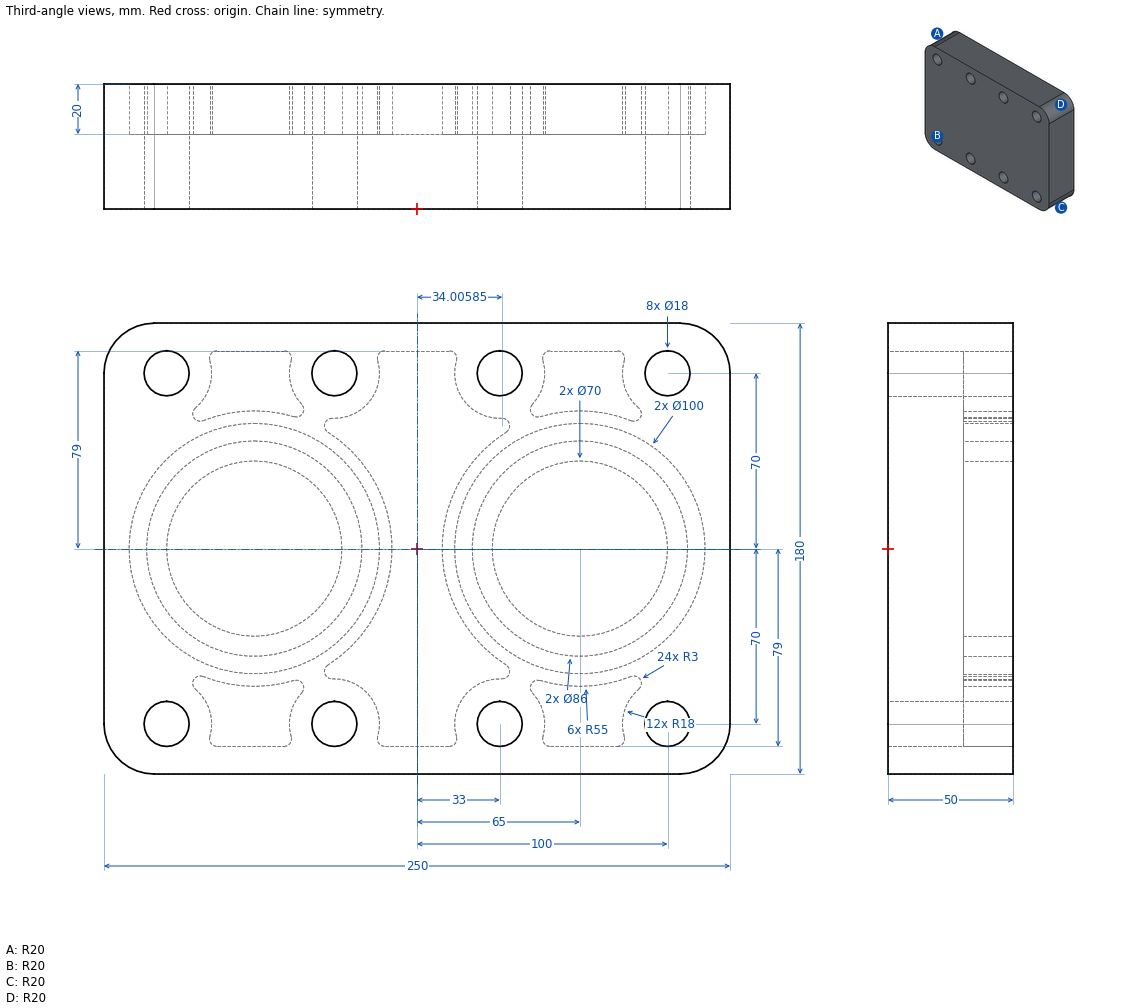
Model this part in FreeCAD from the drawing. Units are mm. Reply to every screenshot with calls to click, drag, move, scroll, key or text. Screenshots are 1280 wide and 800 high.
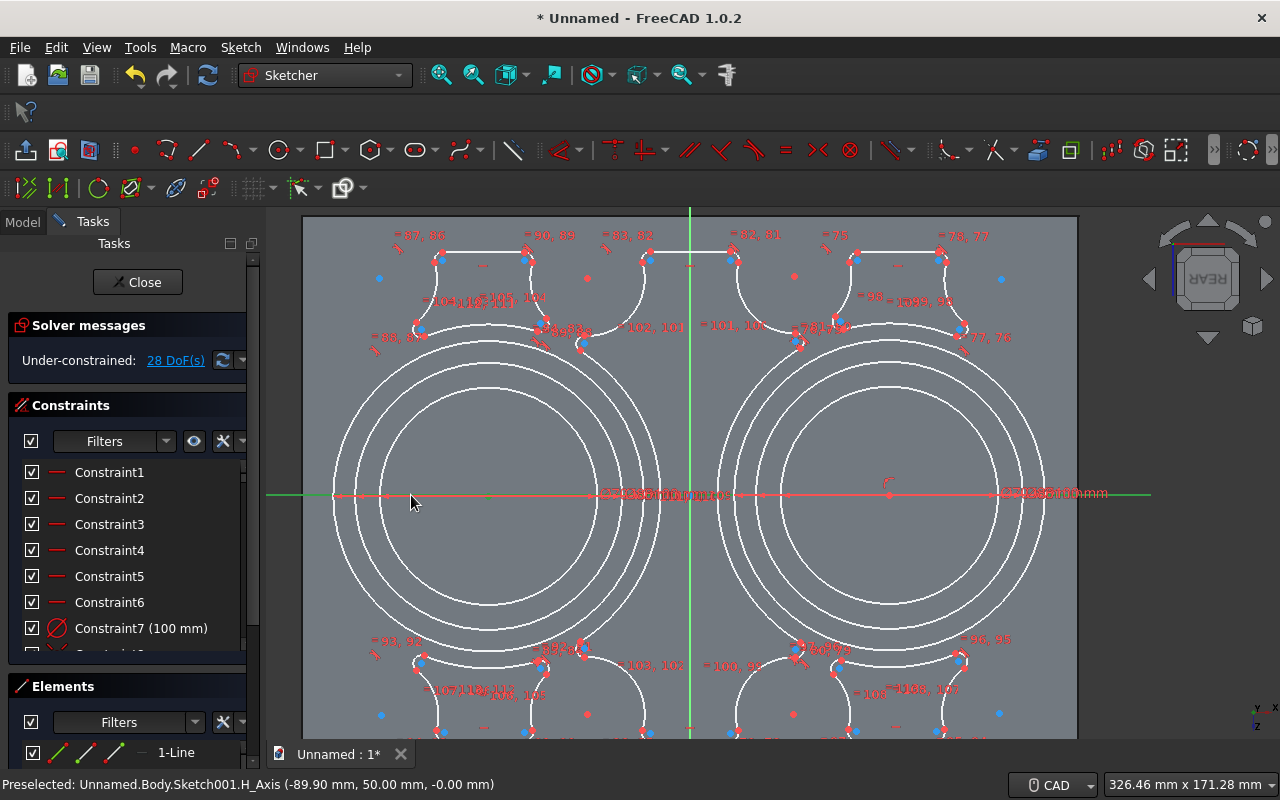
click(614, 150)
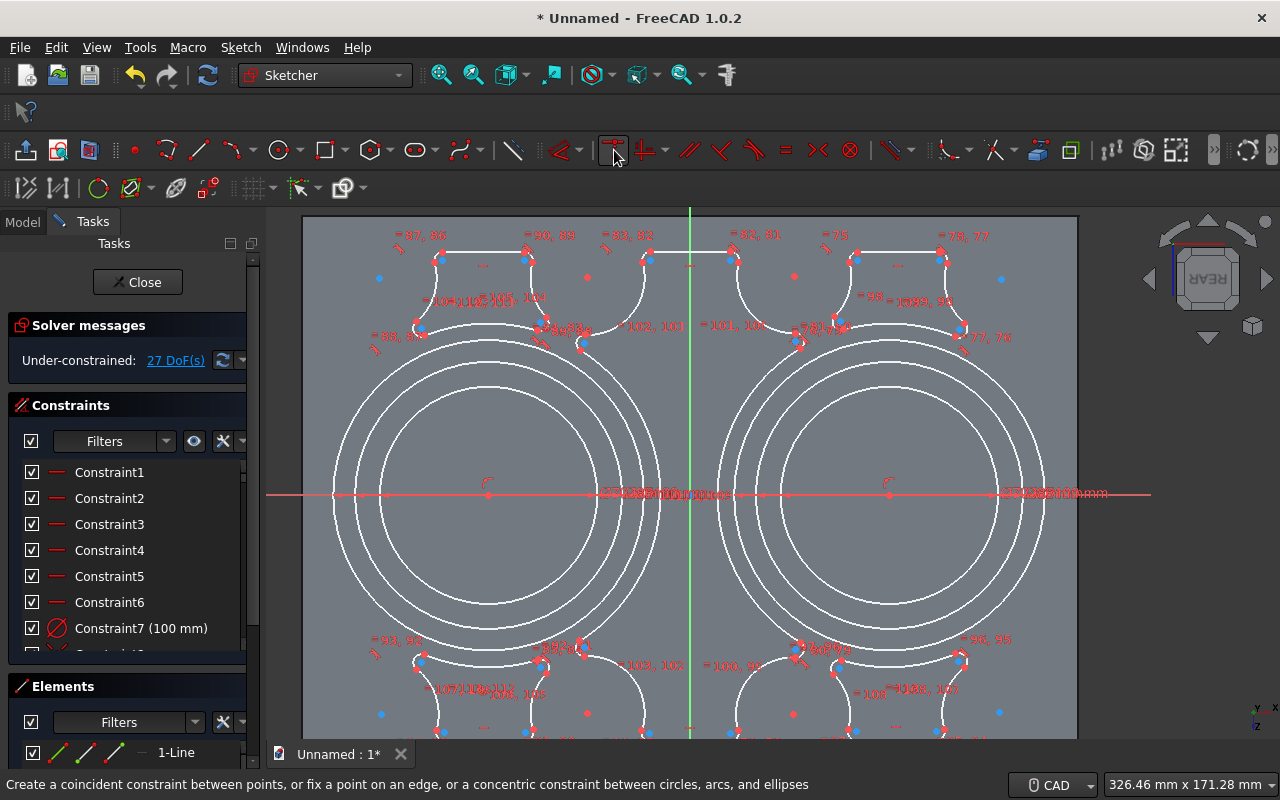
click(794, 276)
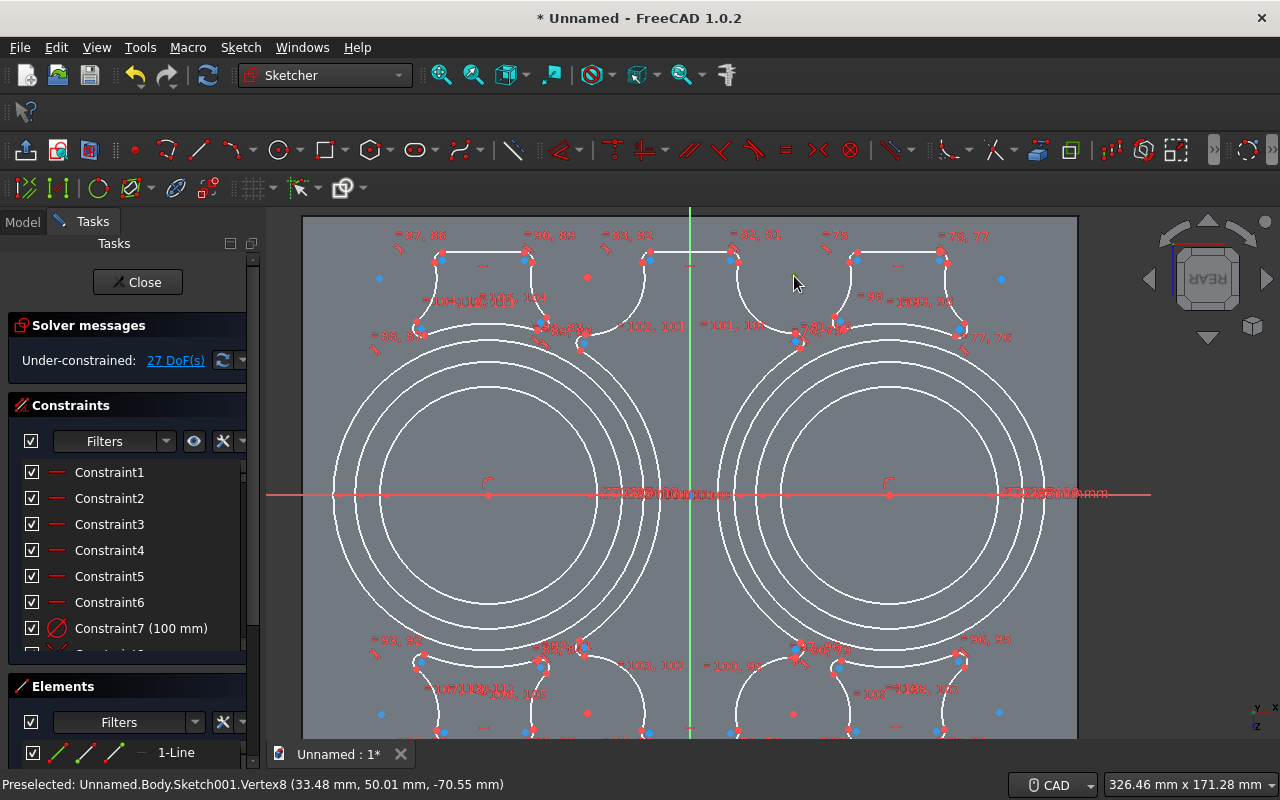
scroll(733, 427, down, 2)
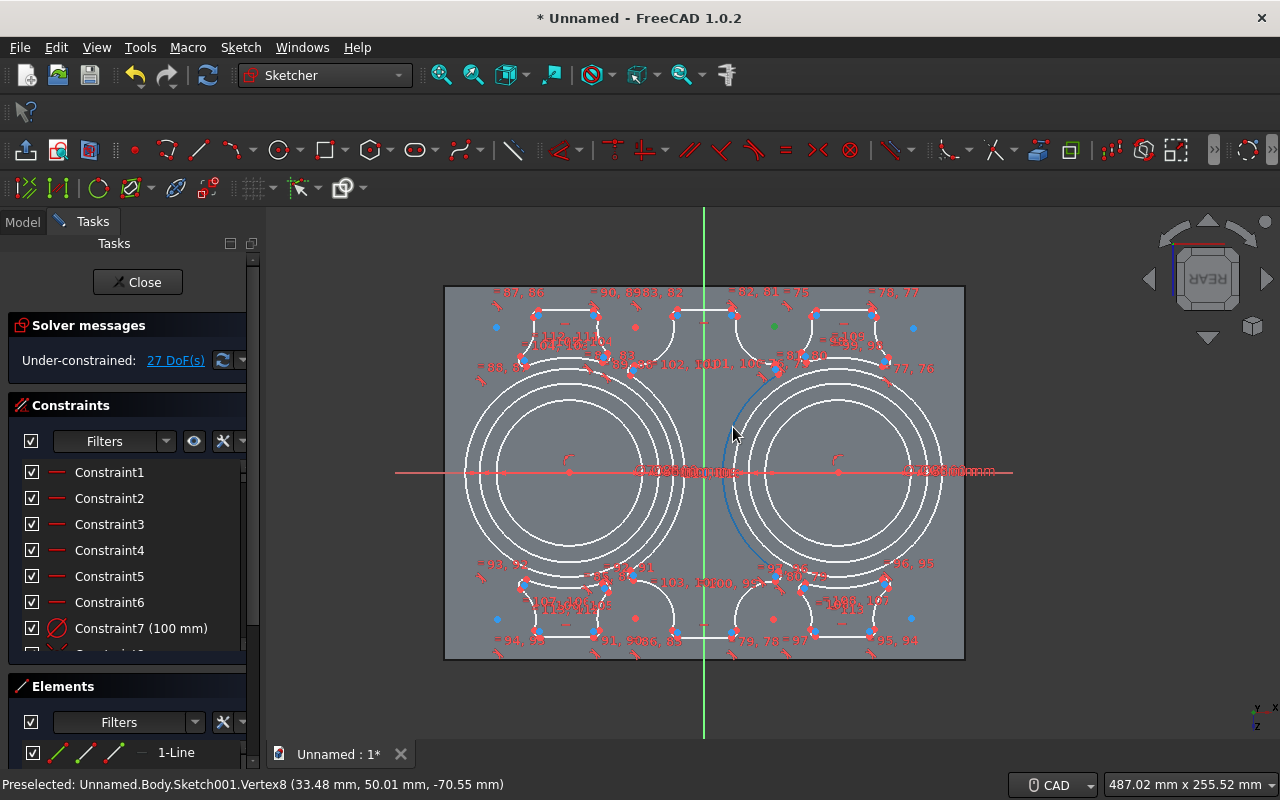
click(773, 620)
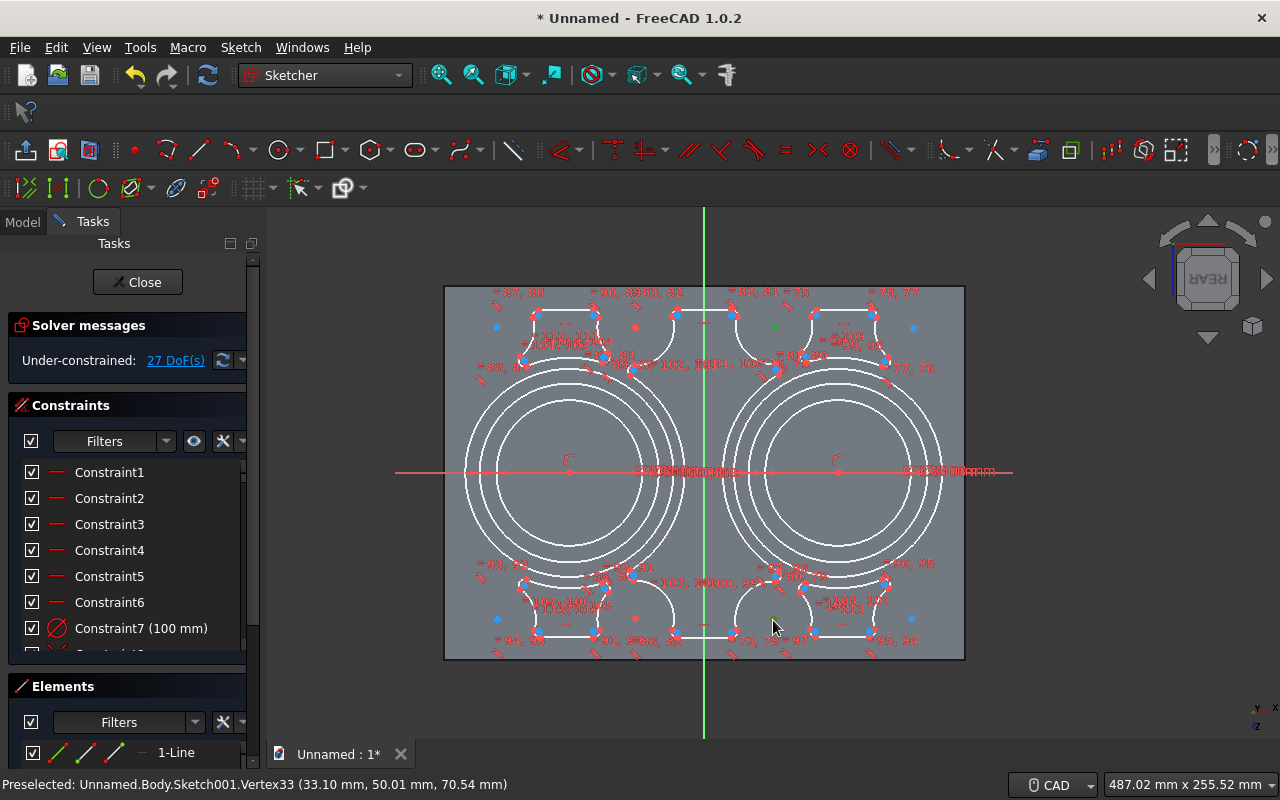
click(411, 473)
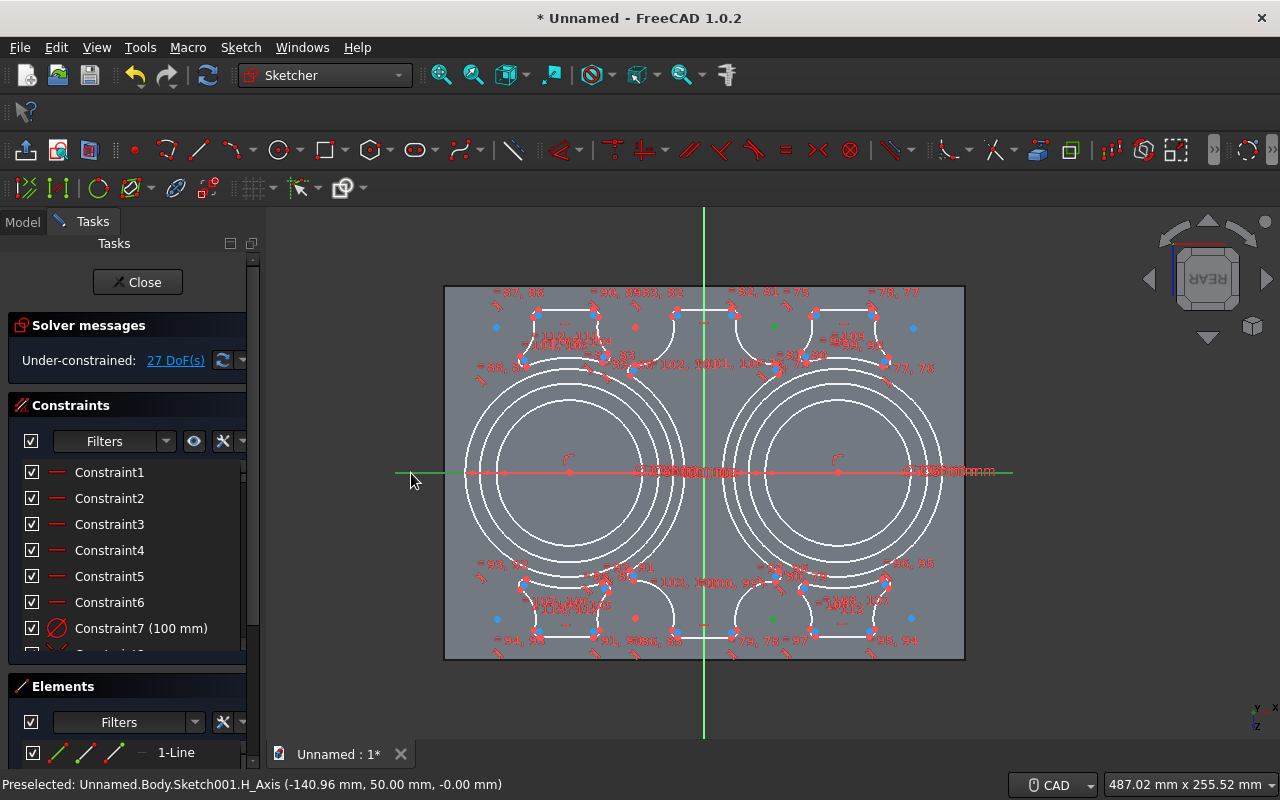
click(818, 150)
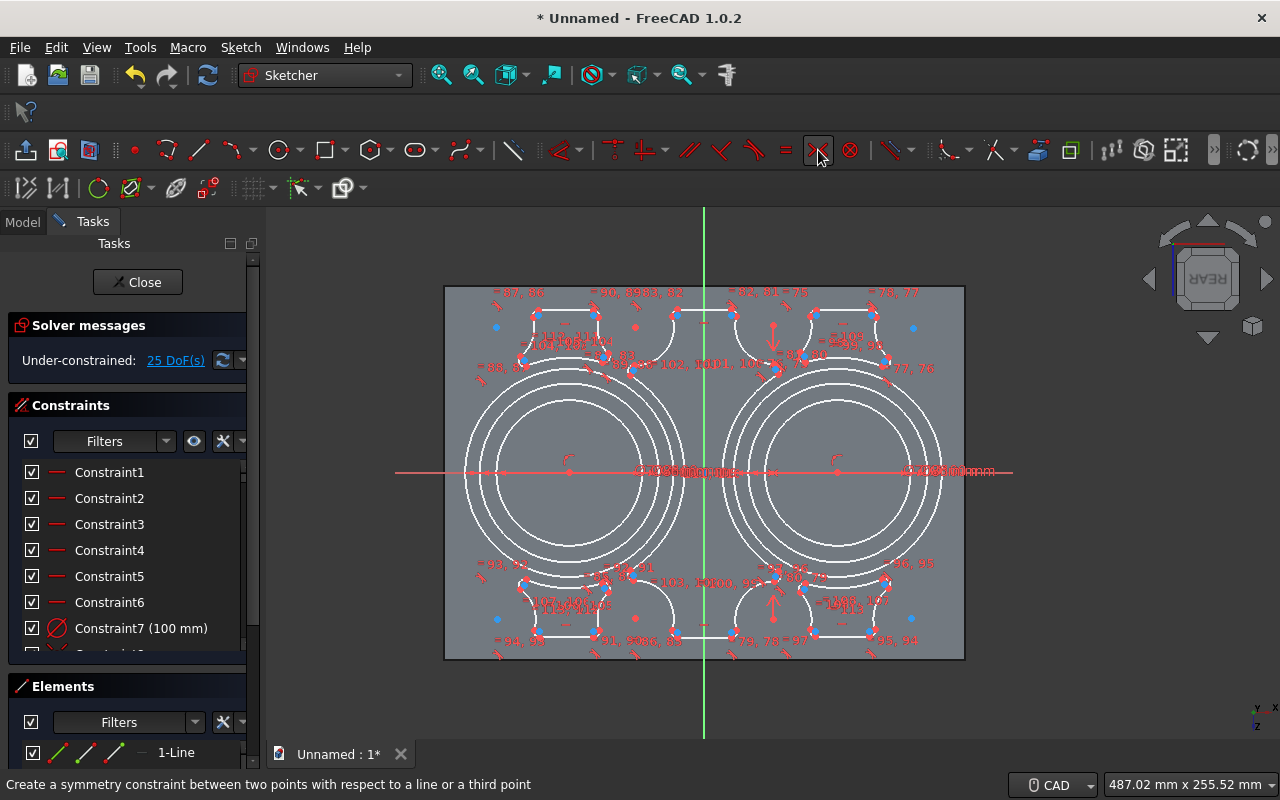
click(773, 326)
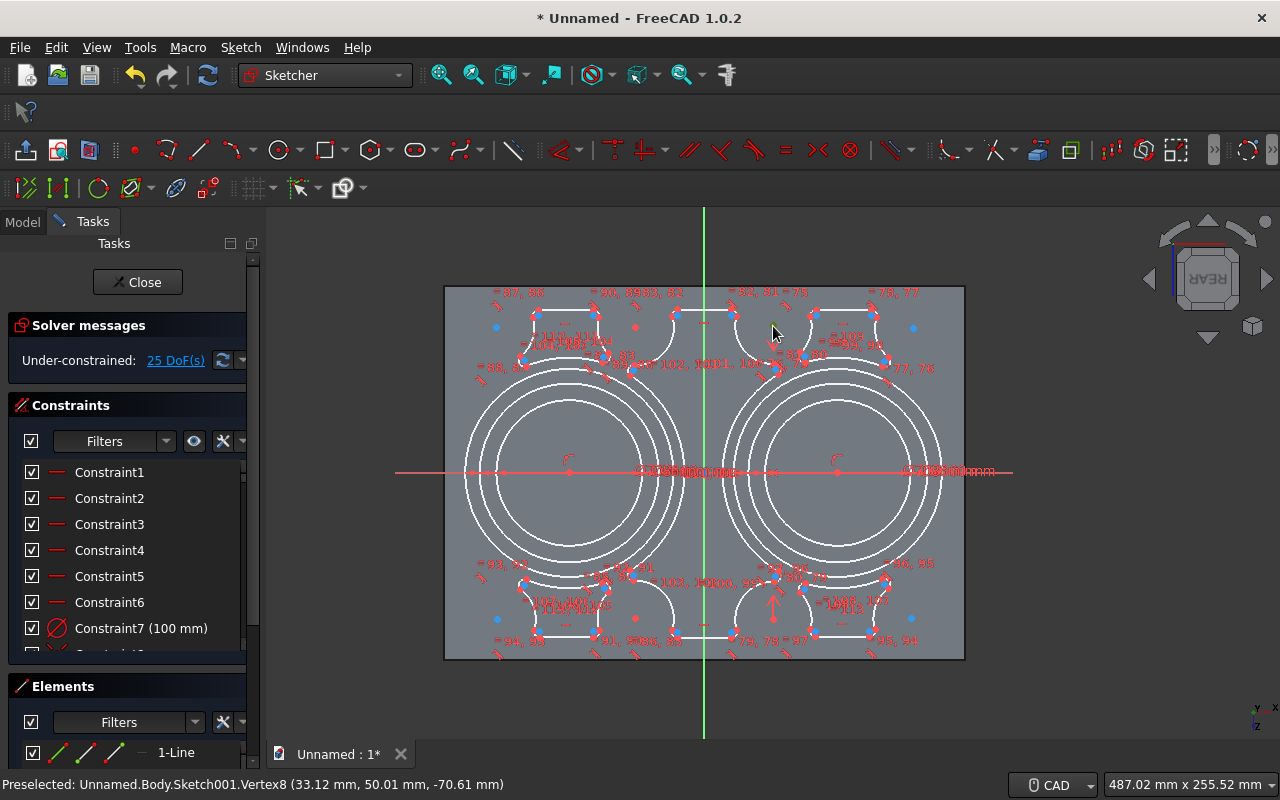
click(636, 327)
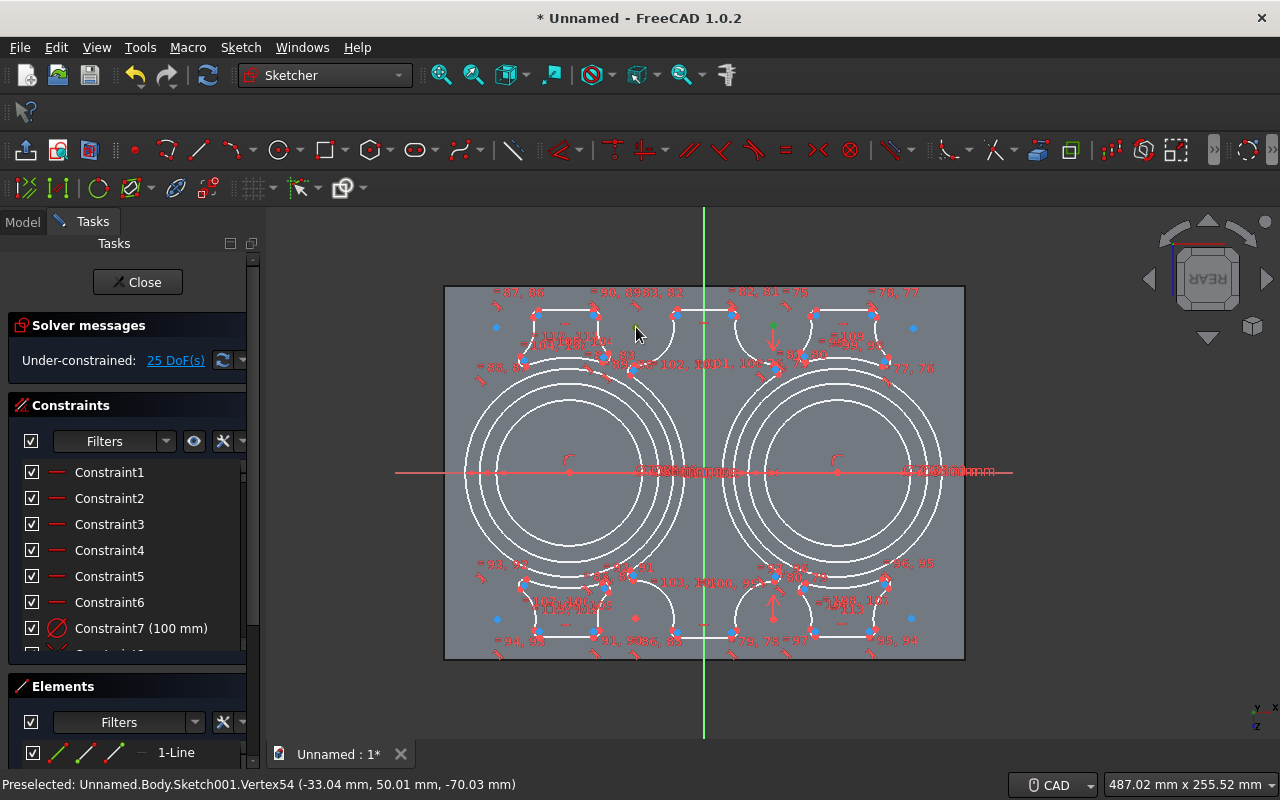
click(704, 677)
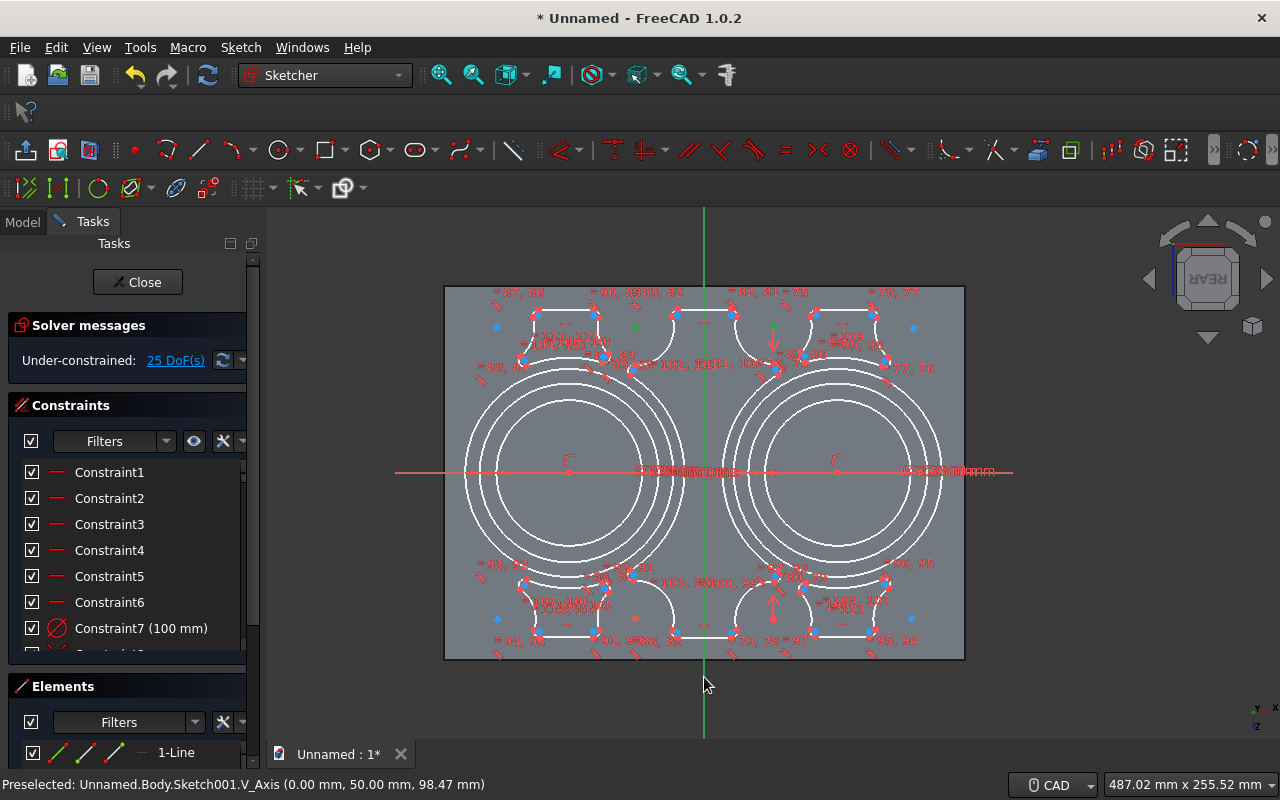
click(818, 150)